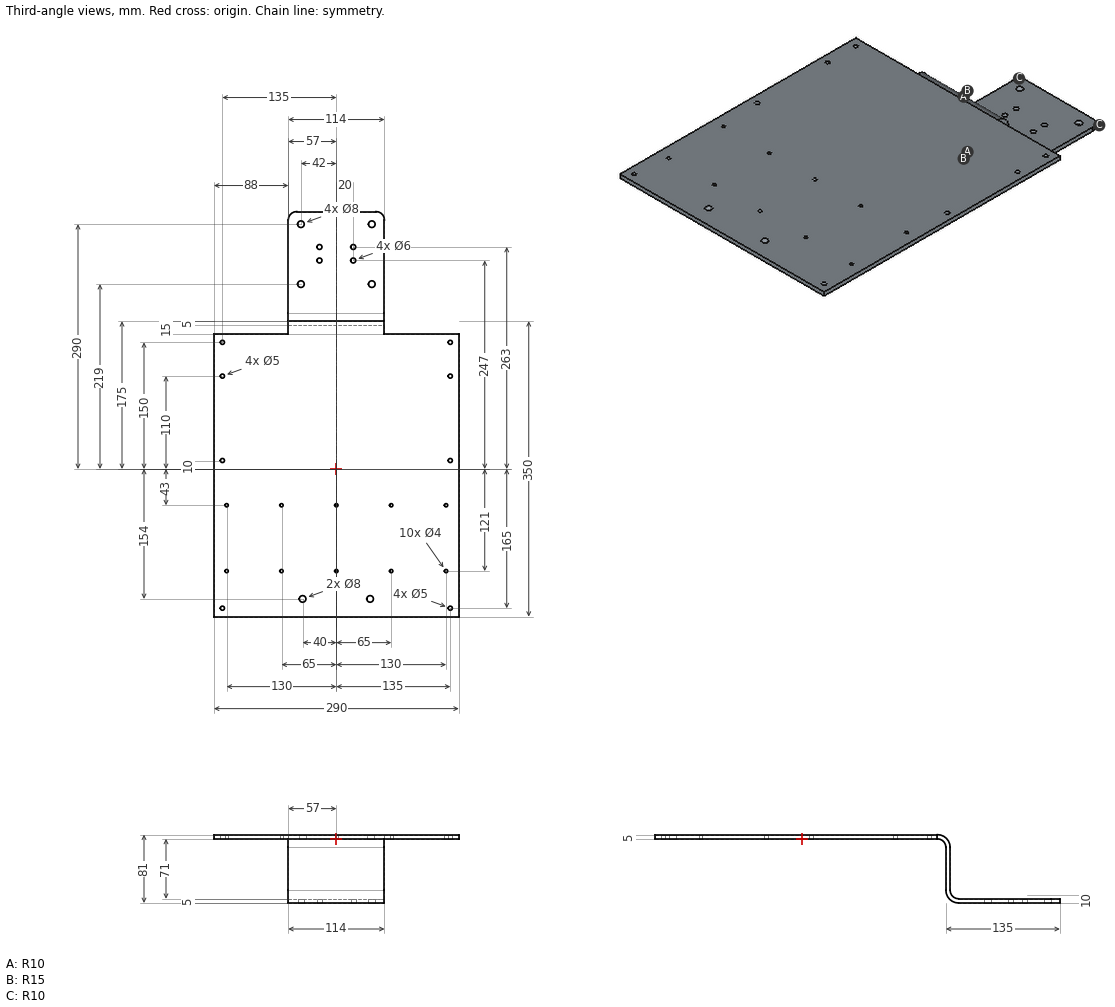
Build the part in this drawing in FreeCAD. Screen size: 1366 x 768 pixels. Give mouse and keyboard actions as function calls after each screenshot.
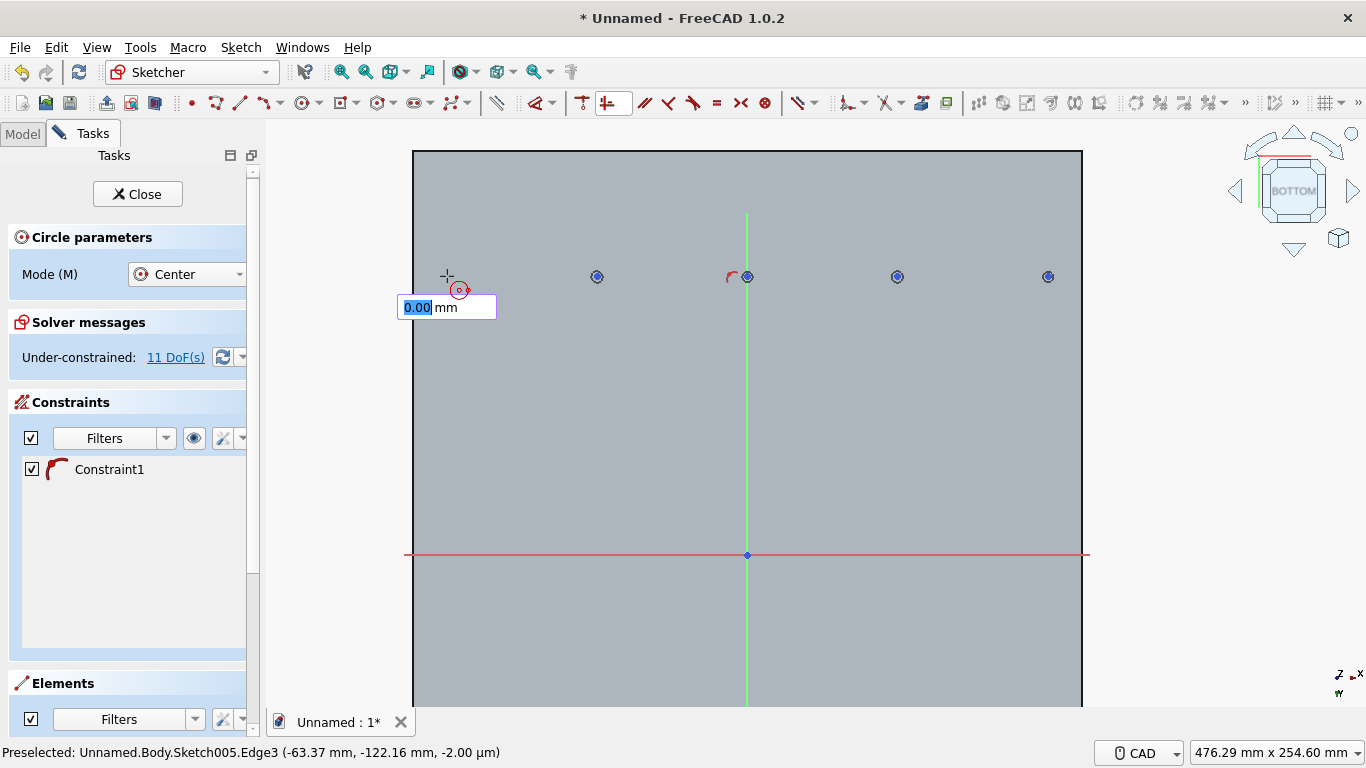
scroll(451, 273, up, 7)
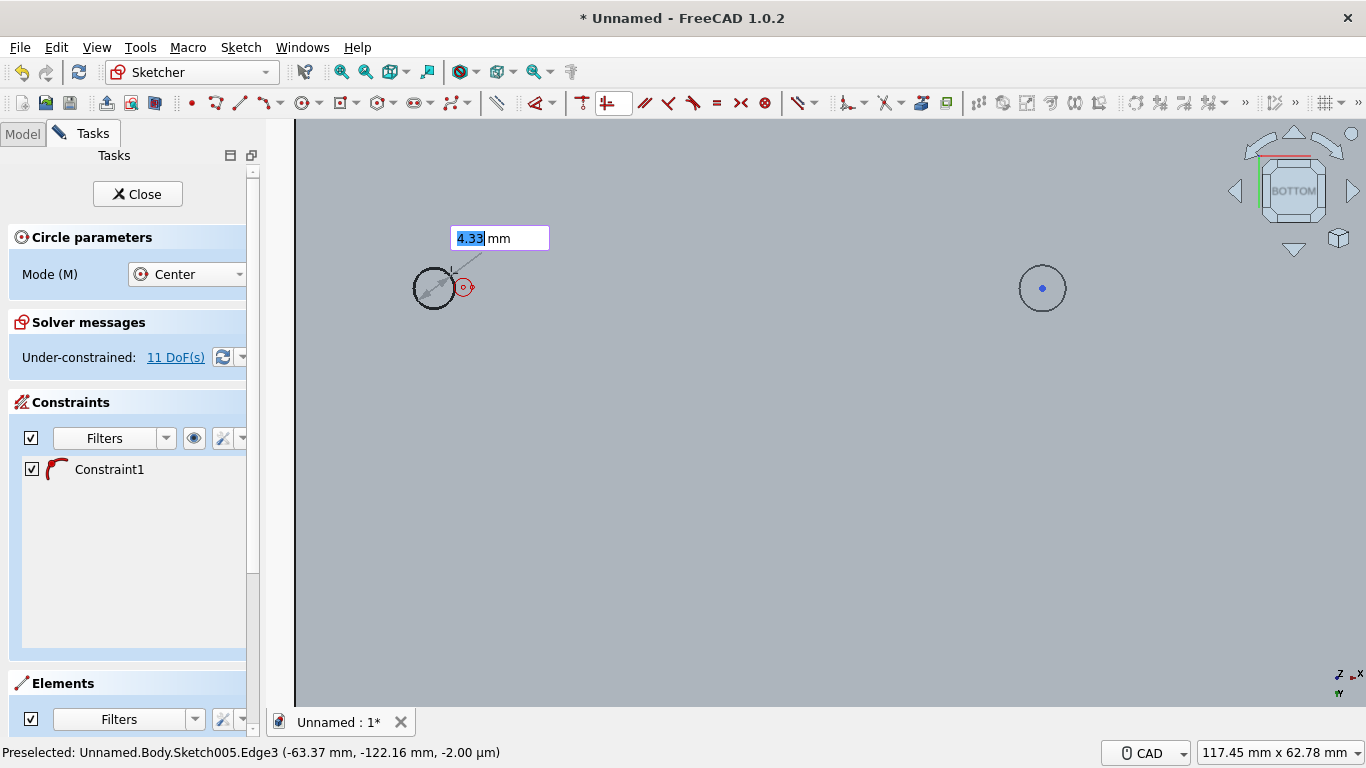
click(449, 270)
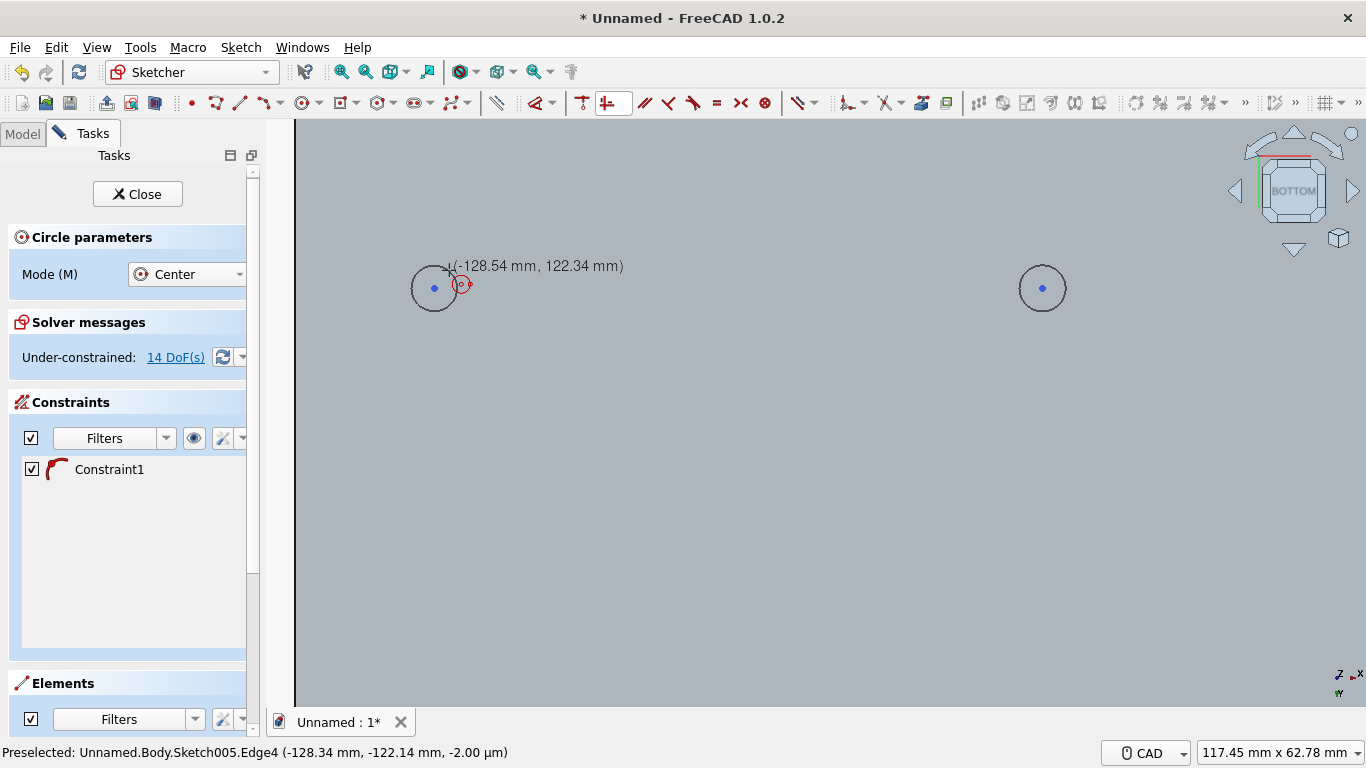
scroll(451, 273, down, 7)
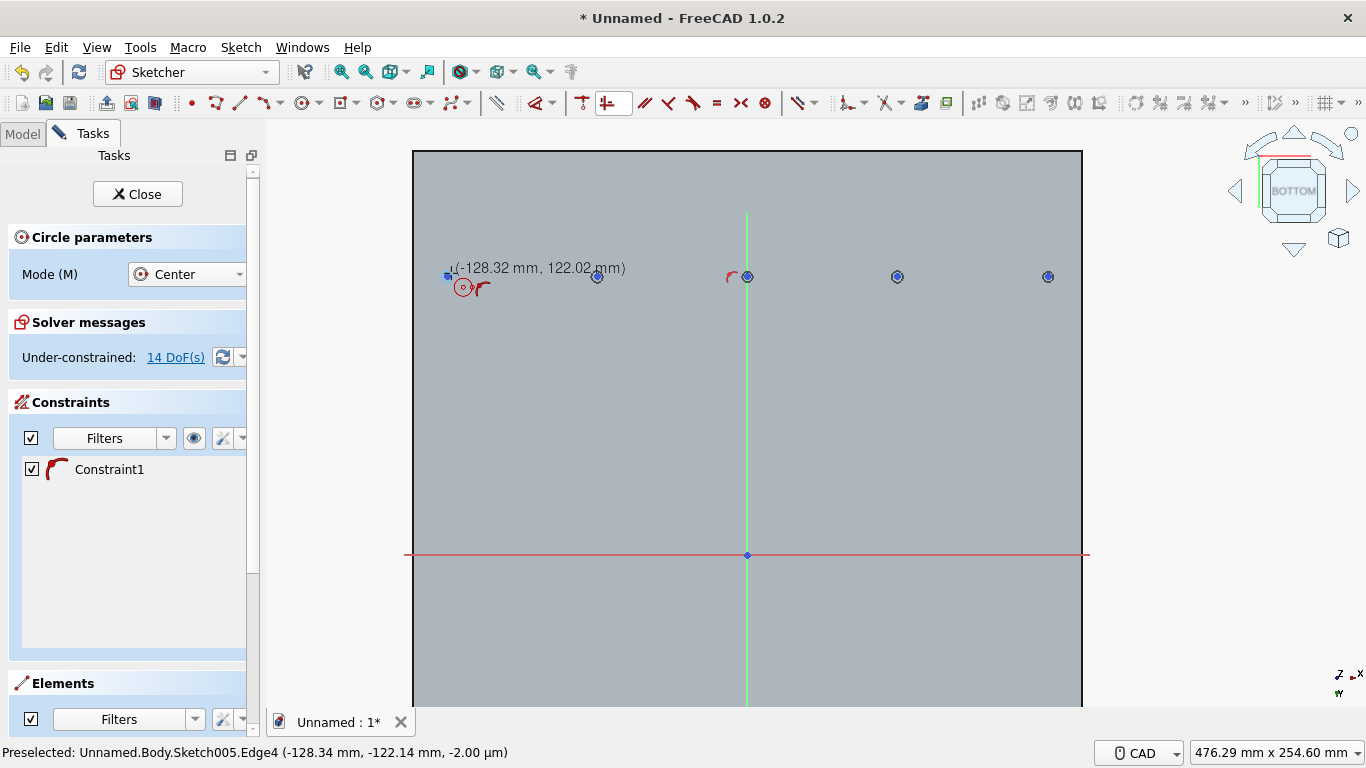
scroll(447, 456, up, 8)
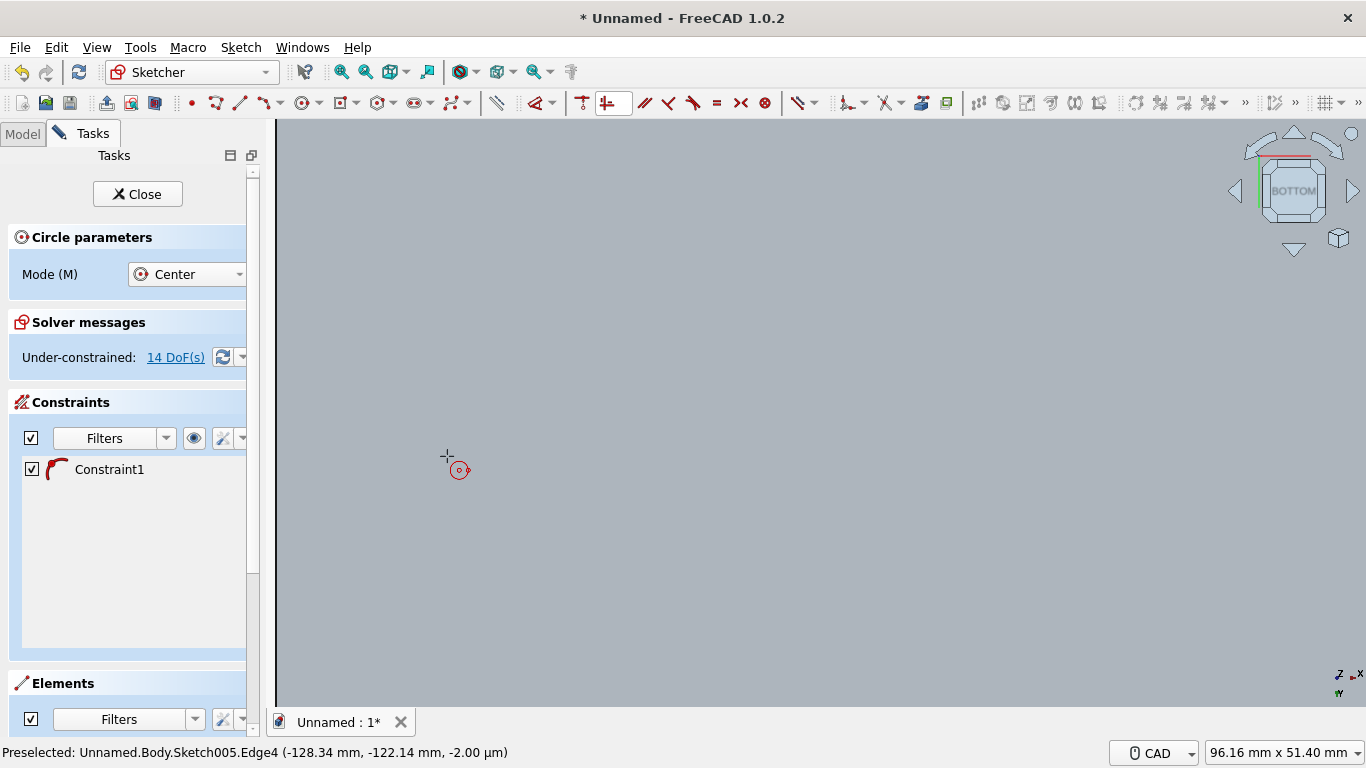
scroll(447, 456, down, 8)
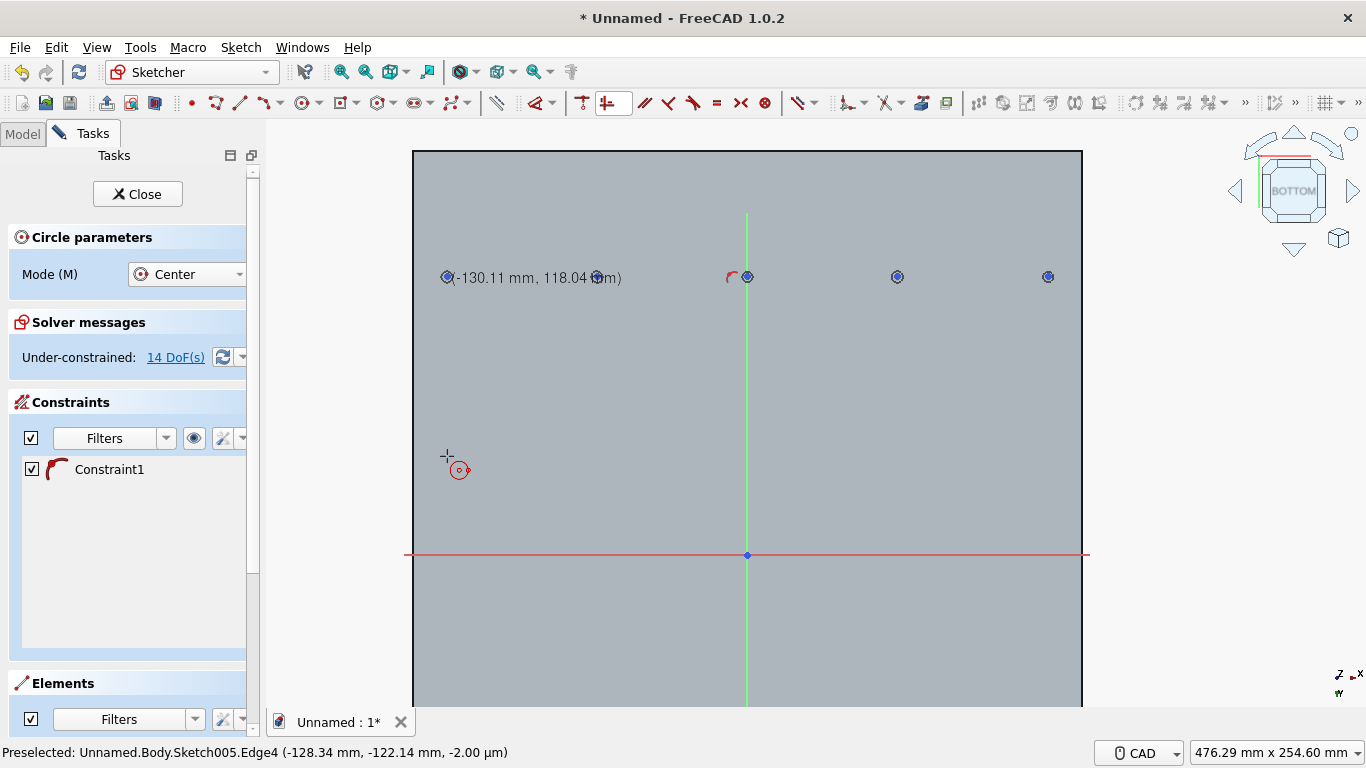
click(447, 456)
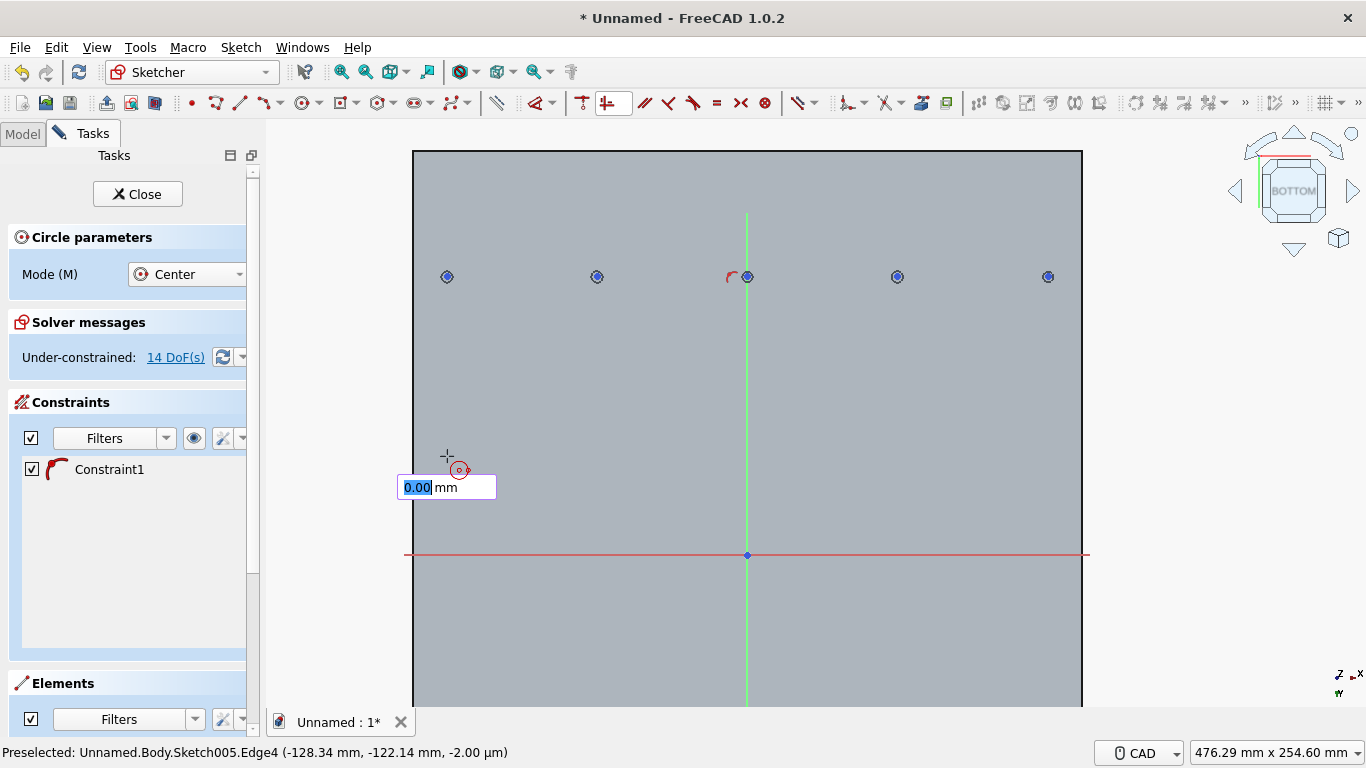
scroll(451, 453, up, 7)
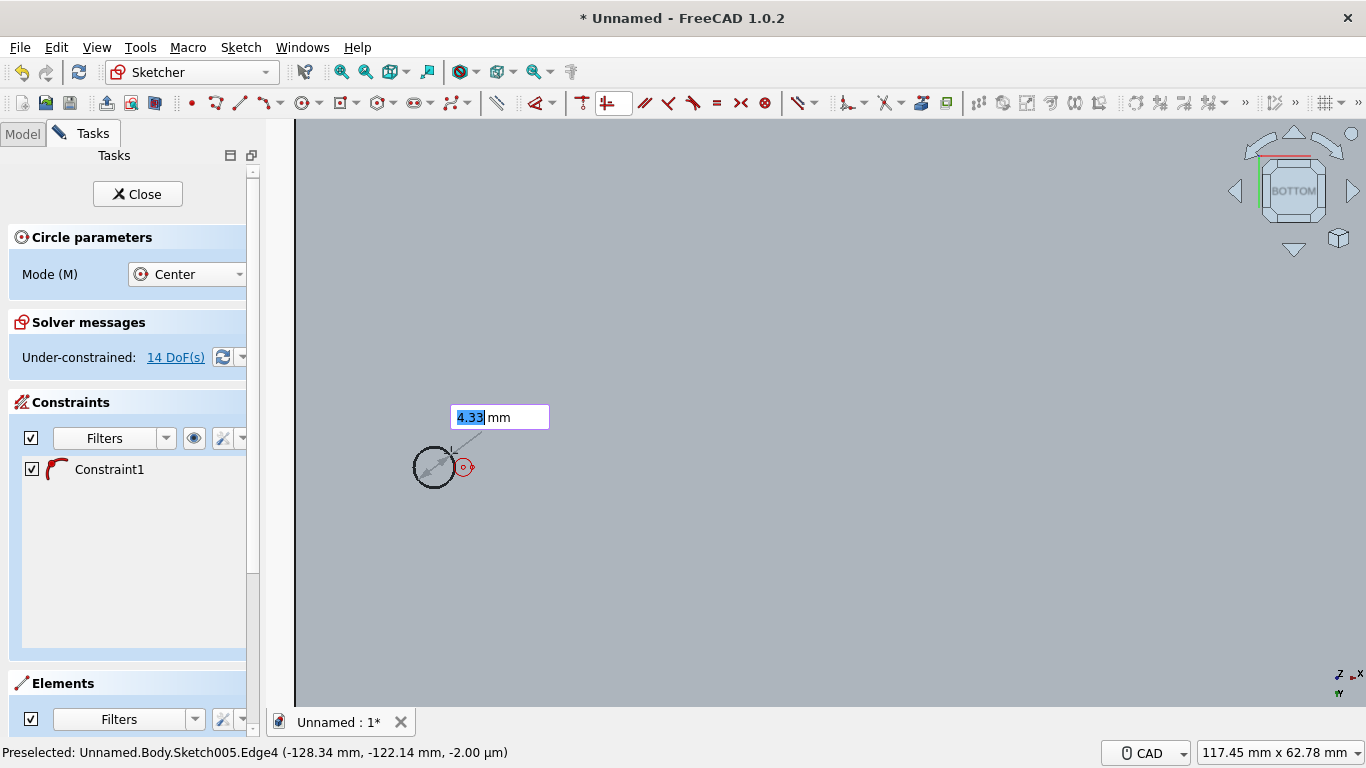
click(449, 450)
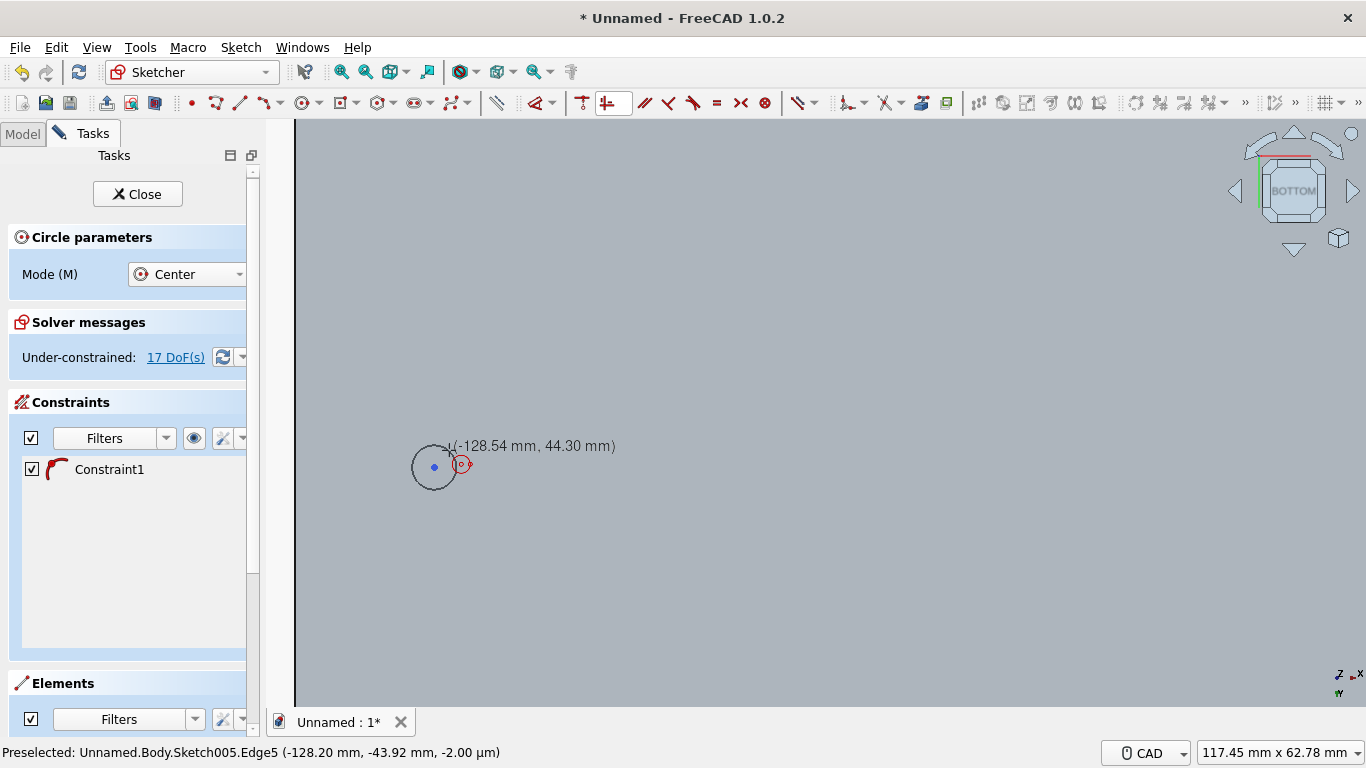
scroll(451, 453, down, 7)